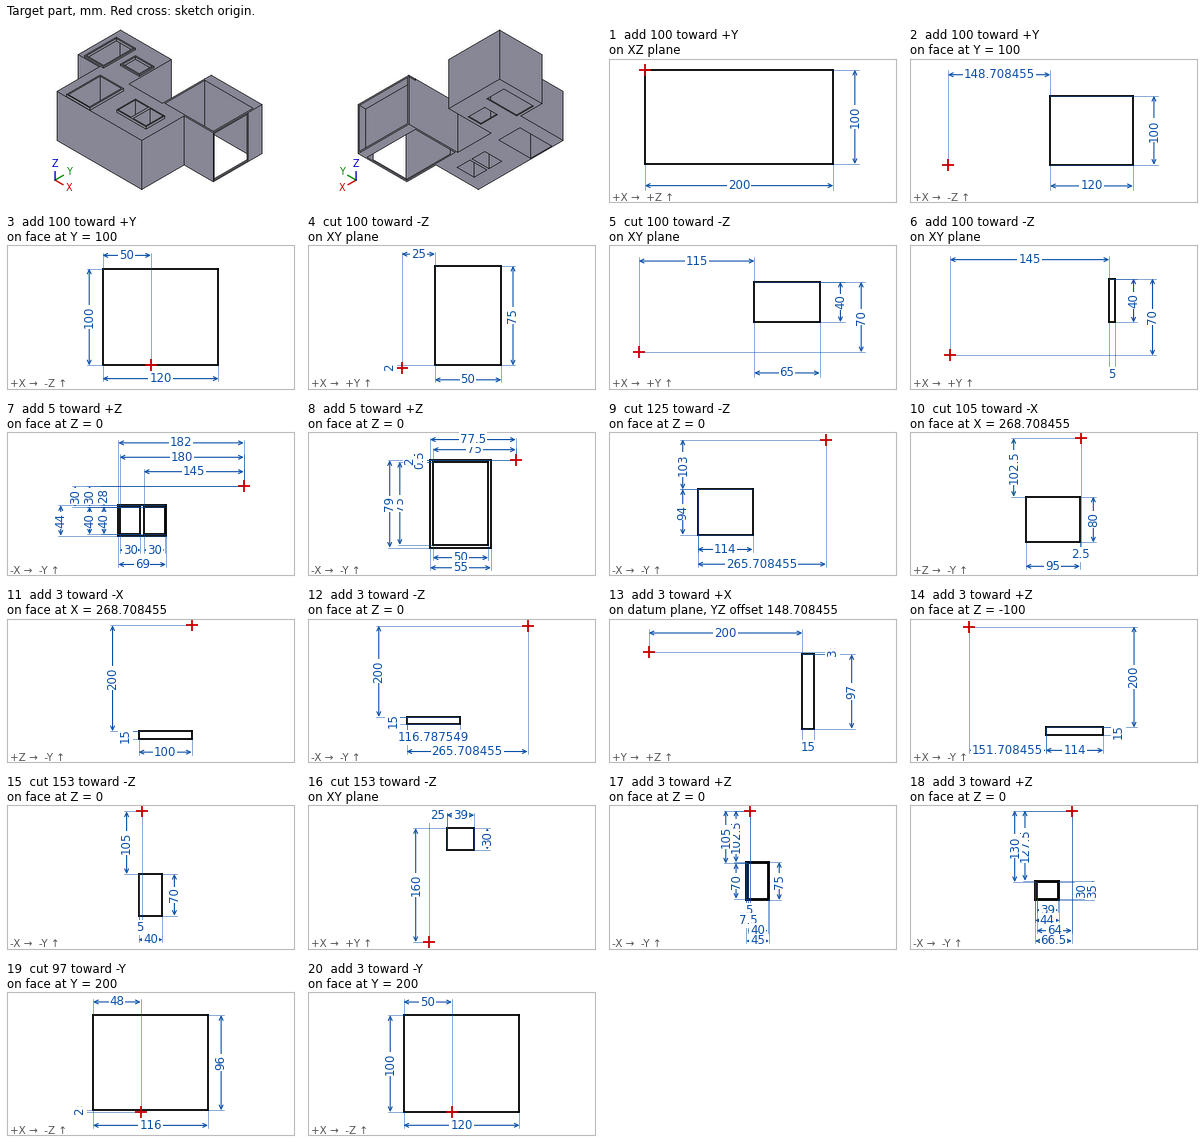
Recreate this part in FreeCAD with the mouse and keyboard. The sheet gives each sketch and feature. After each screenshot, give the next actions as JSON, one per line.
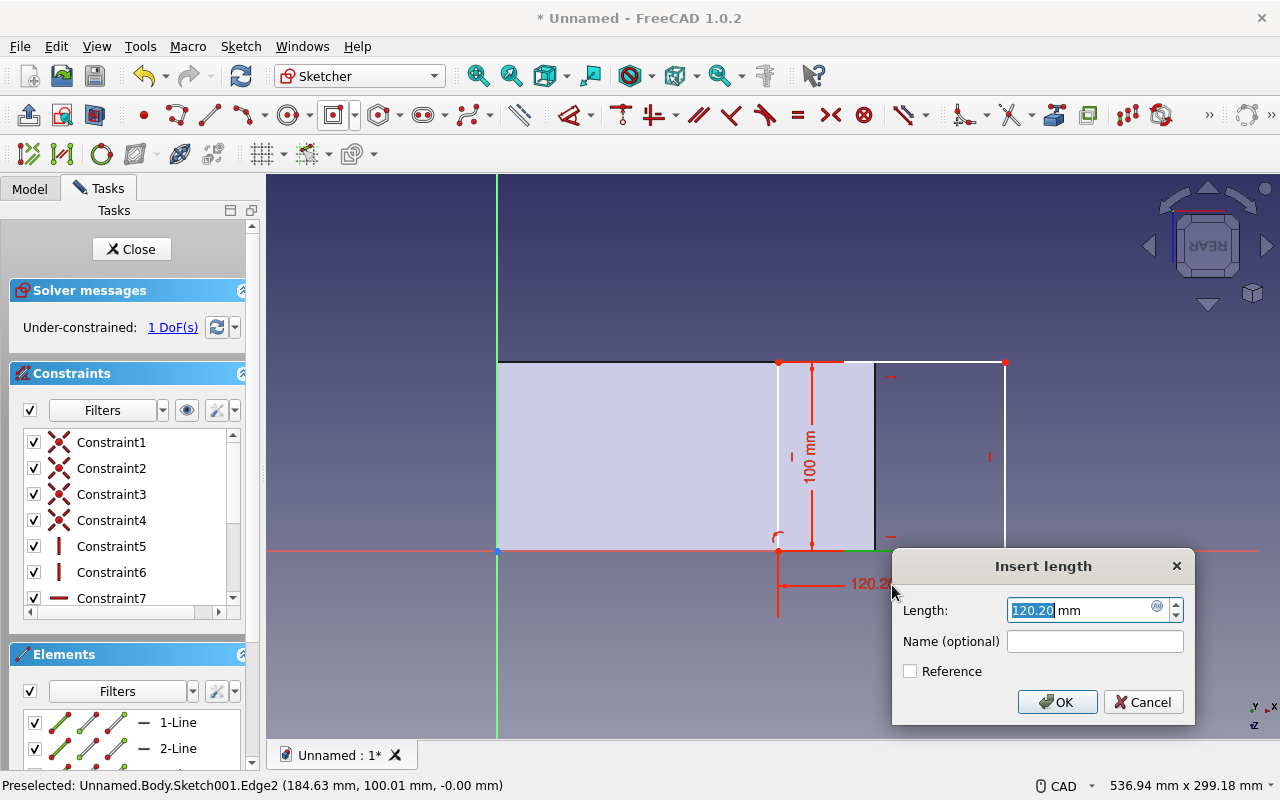
{"action": "type", "text": "120"}
{"action": "key", "text": "Return"}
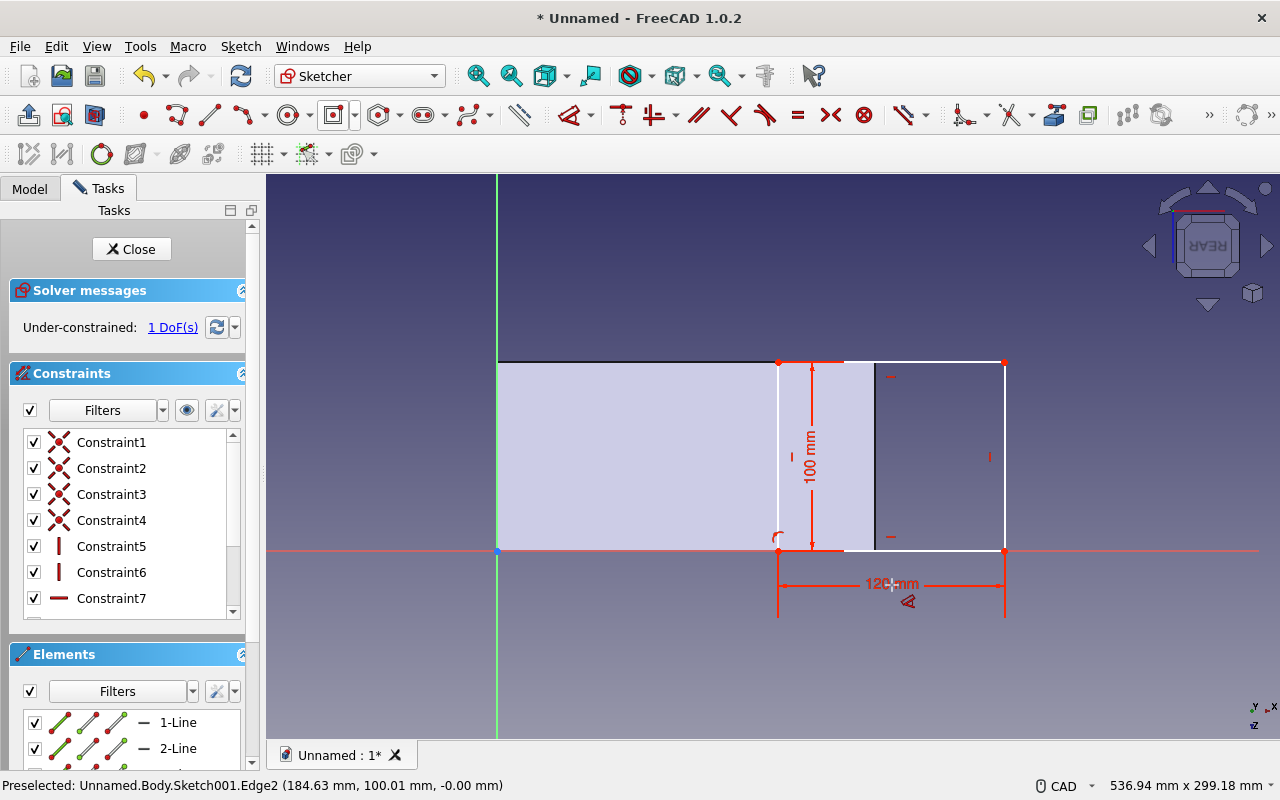
{"action": "left_click", "coordinate": [778, 362]}
{"action": "left_click", "coordinate": [638, 585]}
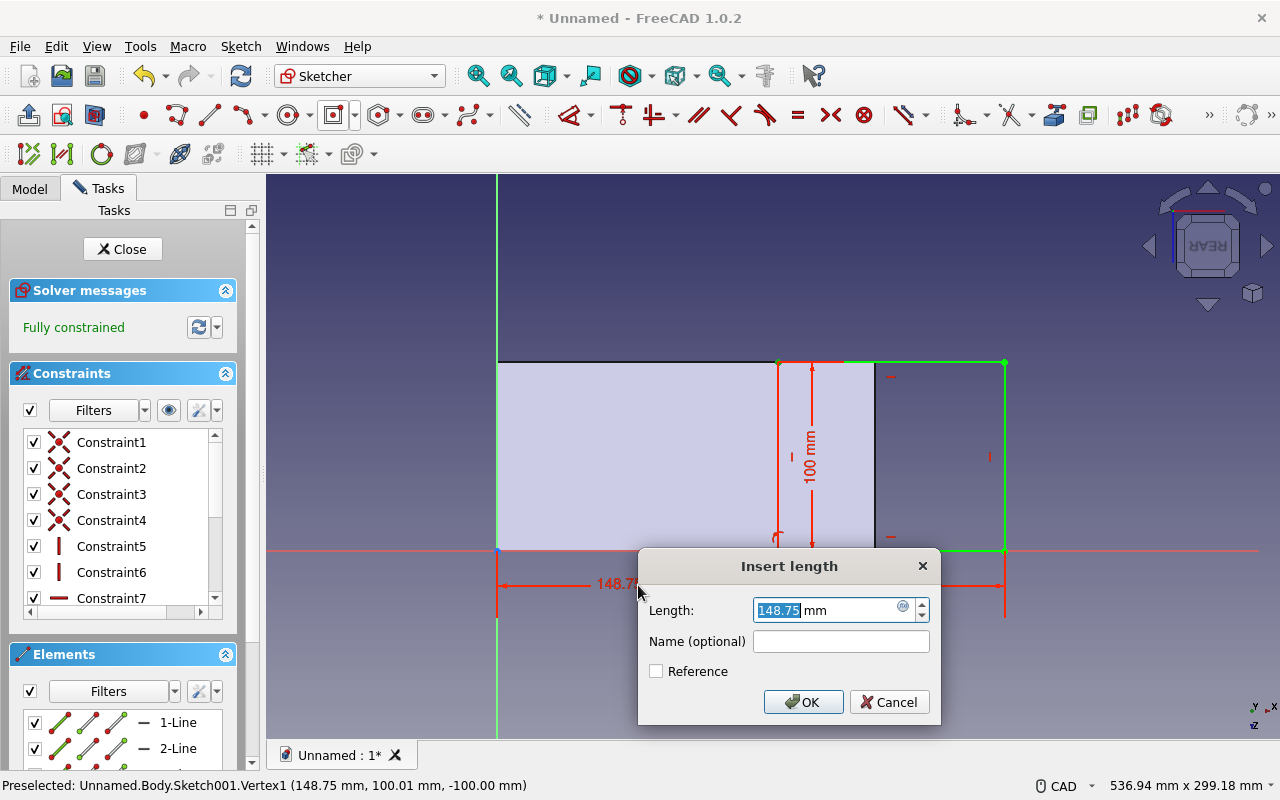
{"action": "type", "text": "148.708455"}
{"action": "key", "text": "Return"}
{"action": "key", "text": "Escape"}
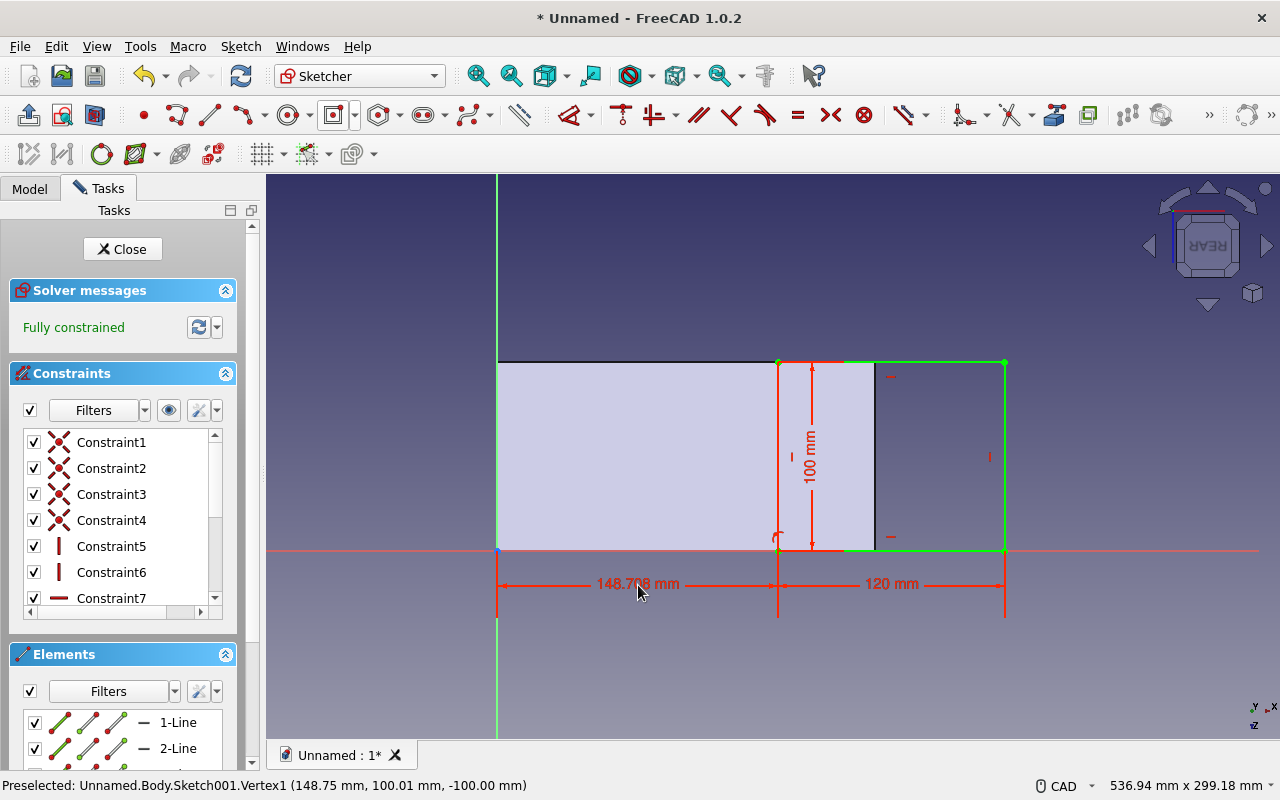
{"action": "left_click", "coordinate": [123, 249]}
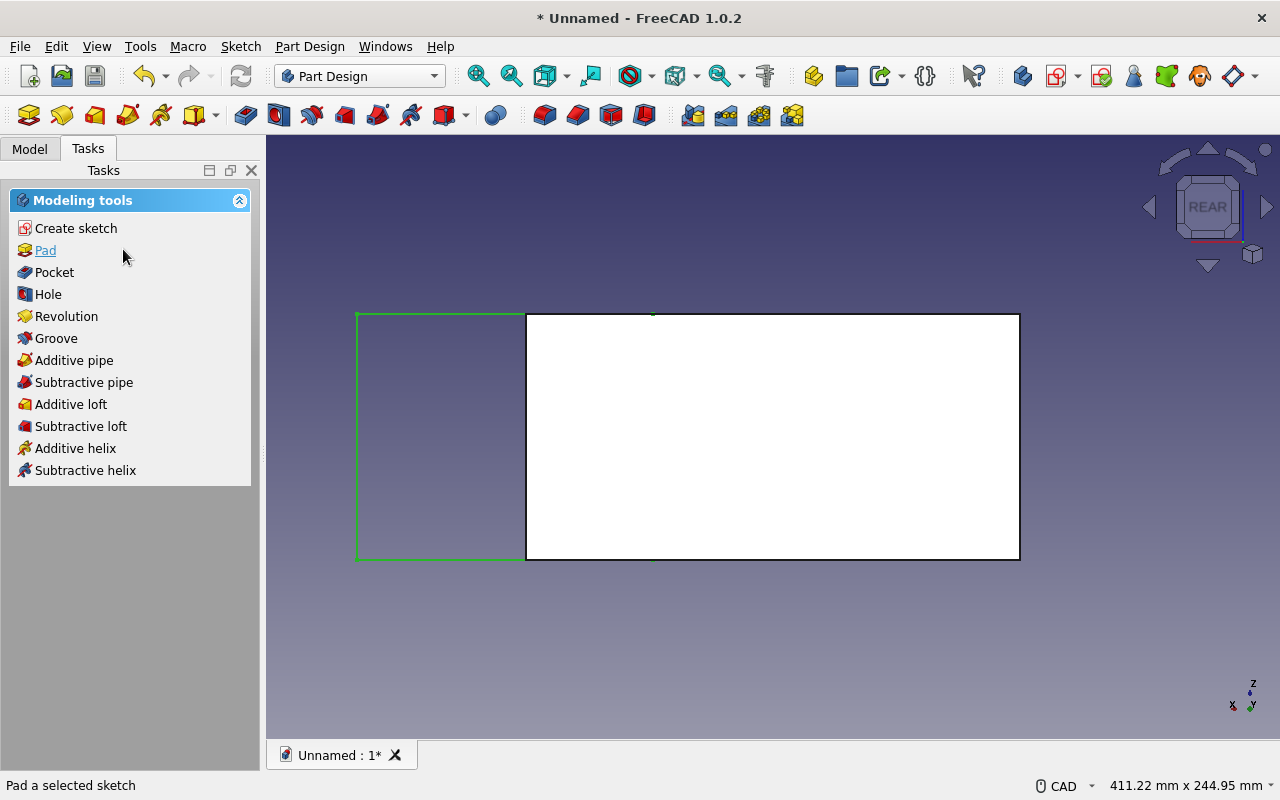
{"action": "left_click", "coordinate": [29, 116]}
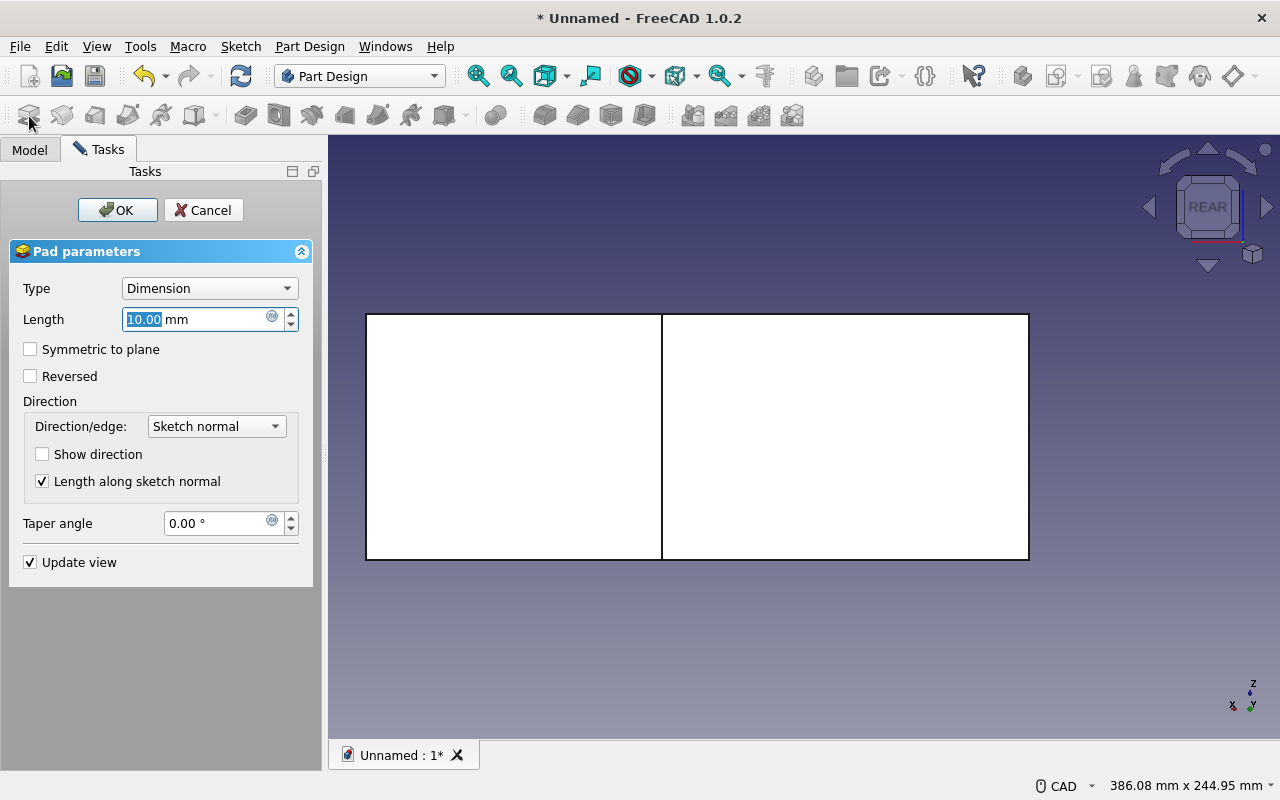
{"action": "type", "text": "100"}
{"action": "key", "text": "Tab"}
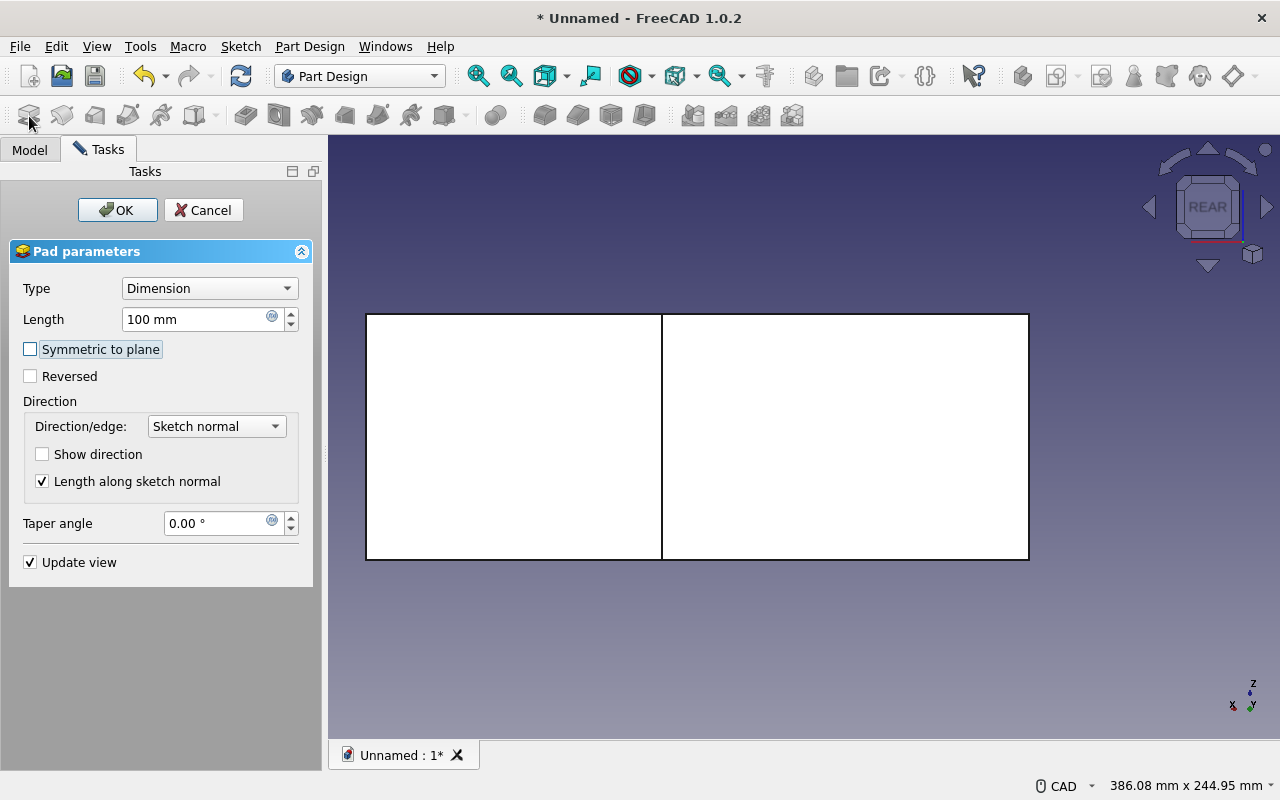
{"action": "left_click", "coordinate": [118, 210]}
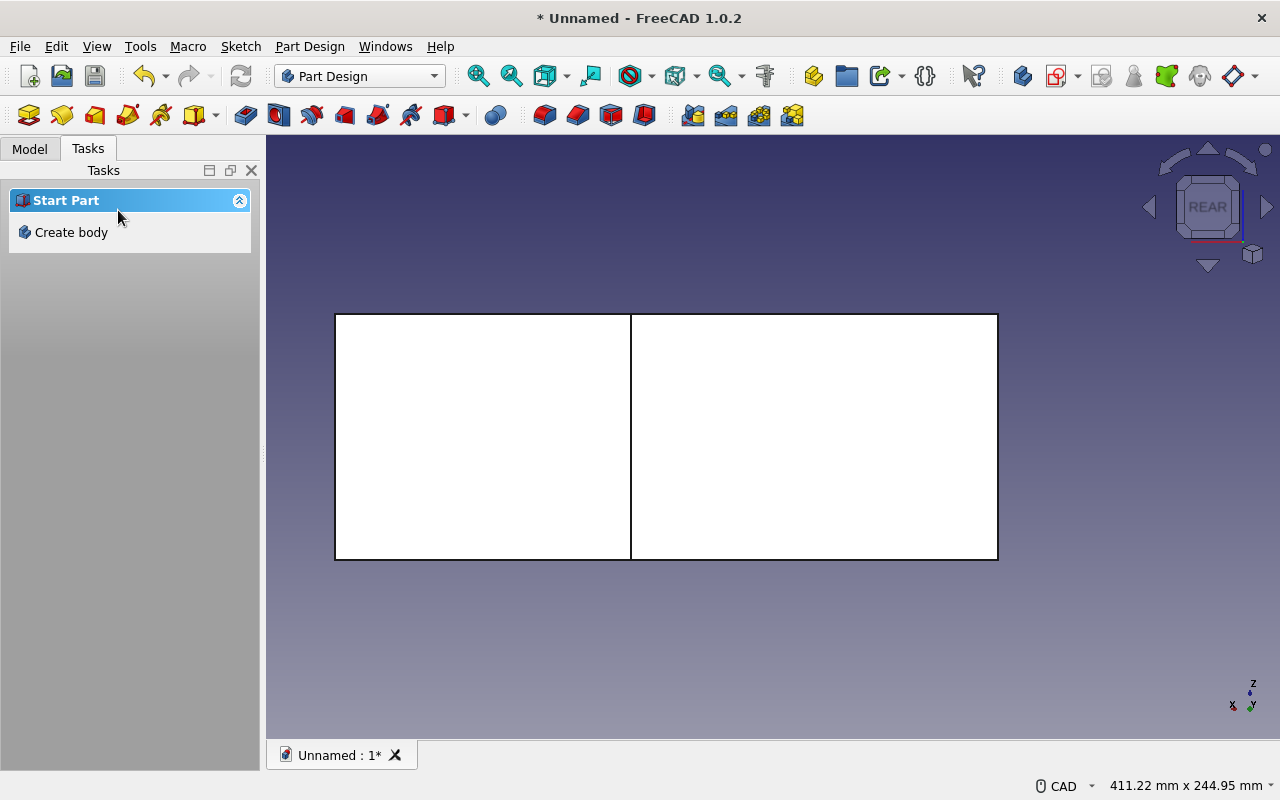
{"action": "left_click", "coordinate": [762, 436]}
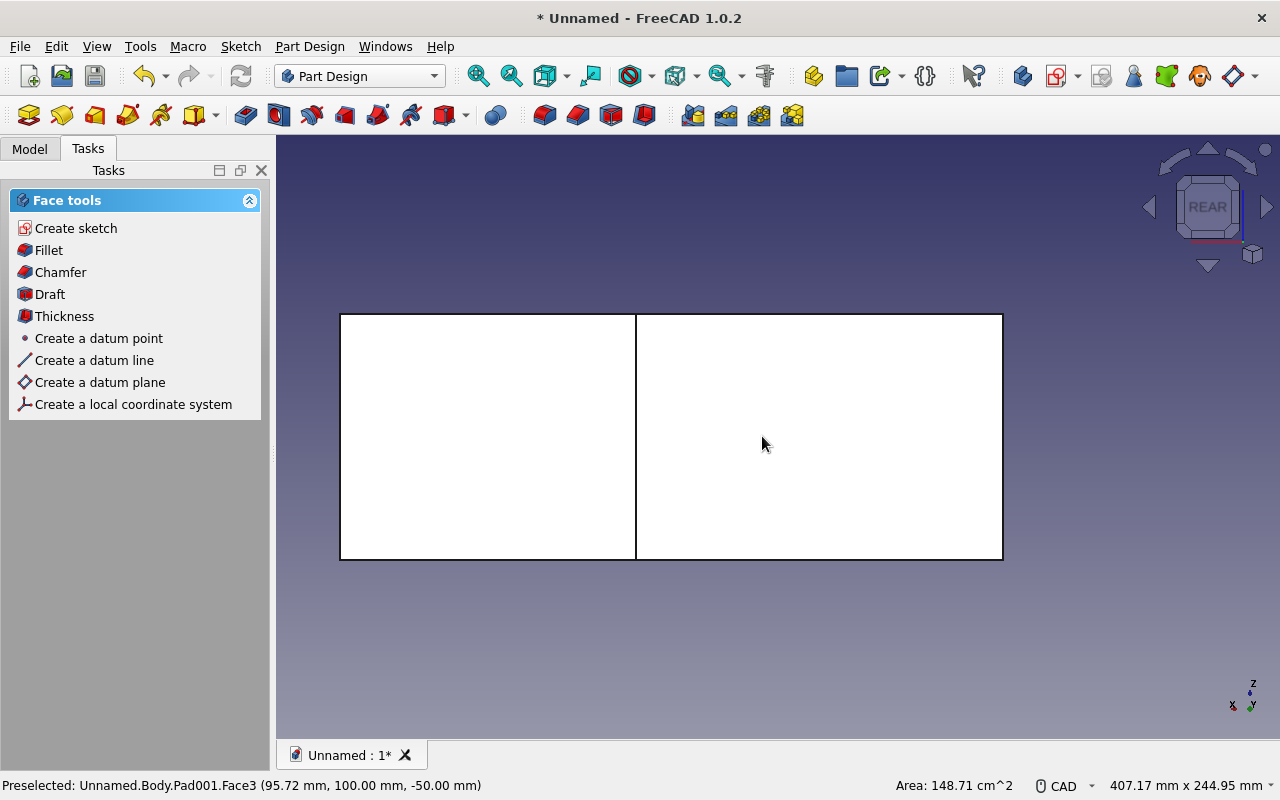
{"action": "left_click", "coordinate": [1056, 76]}